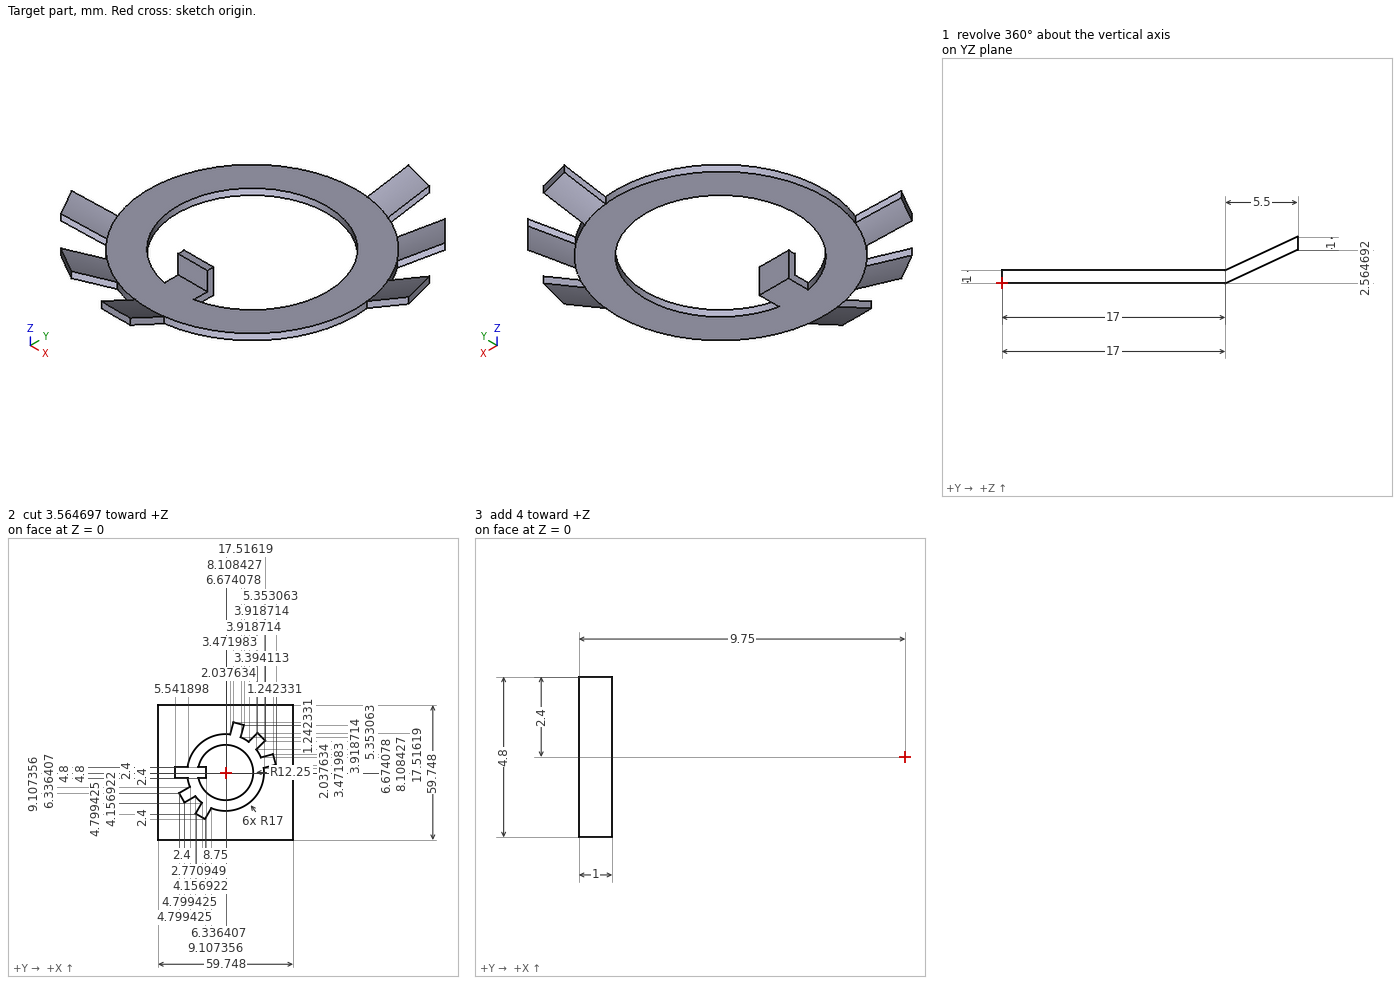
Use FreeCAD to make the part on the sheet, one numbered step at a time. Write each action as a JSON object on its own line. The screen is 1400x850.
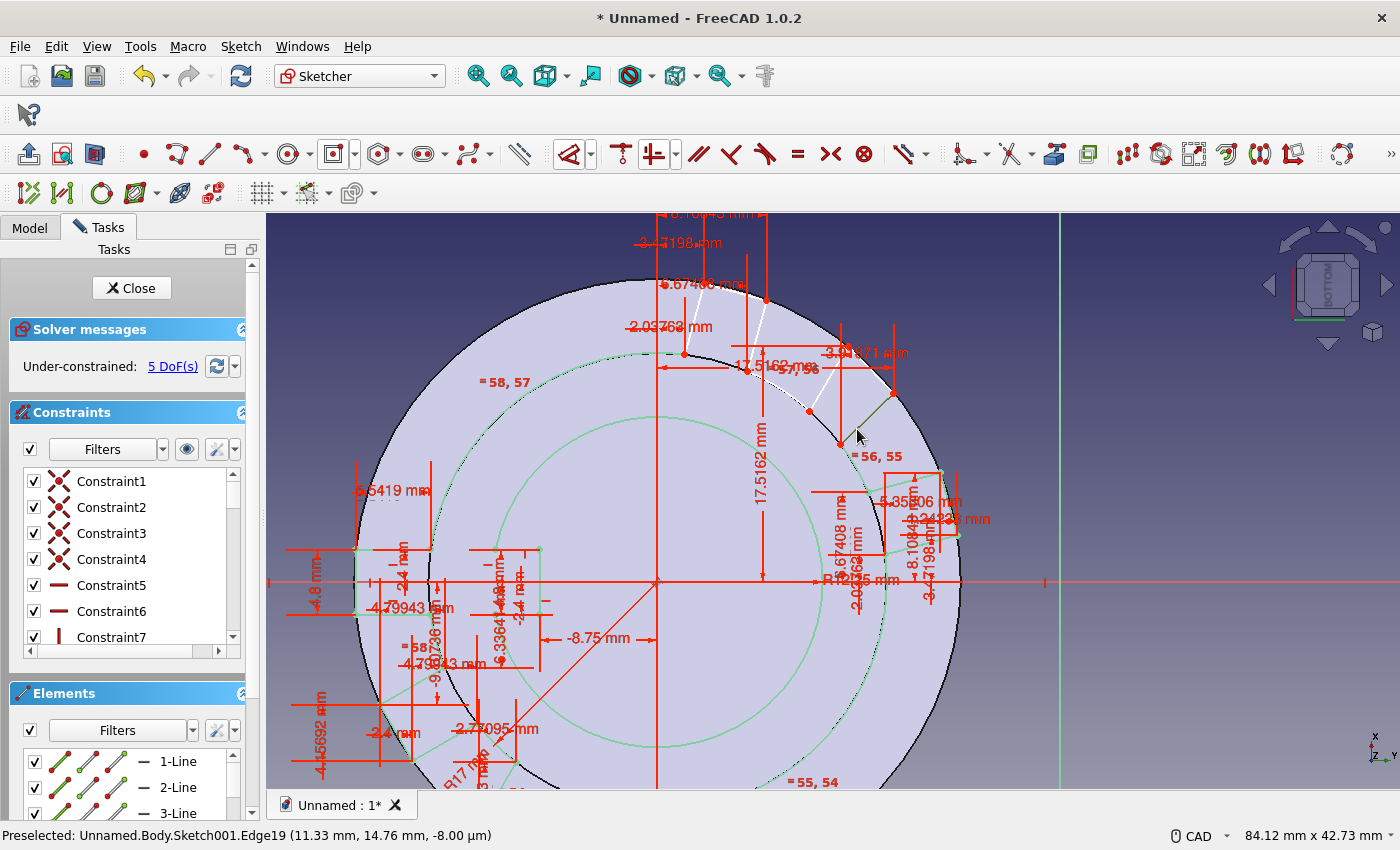
{"action": "key", "text": "i"}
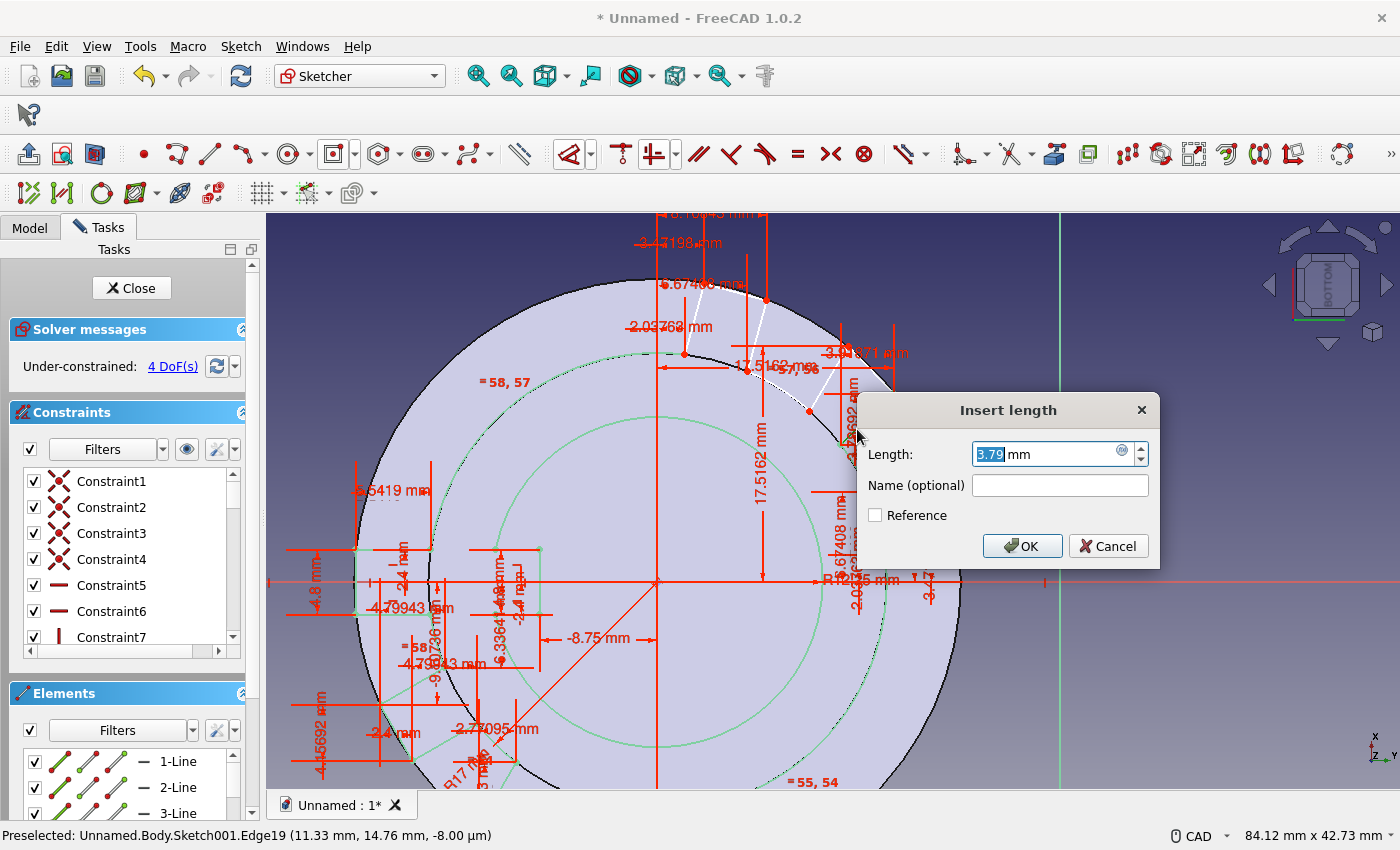
{"action": "type", "text": "3.918714"}
{"action": "key", "text": "Return"}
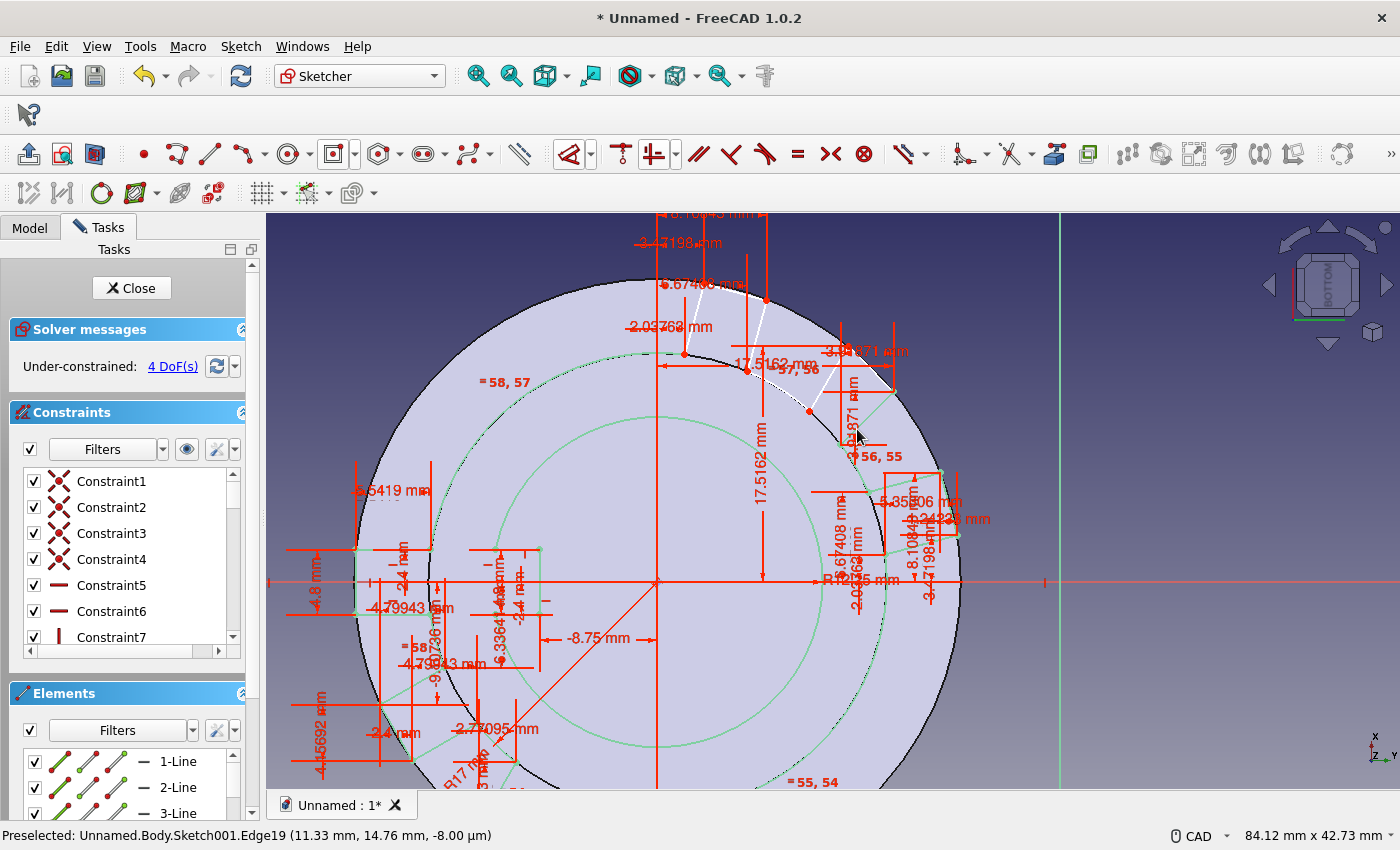
{"action": "left_click", "coordinate": [880, 378]}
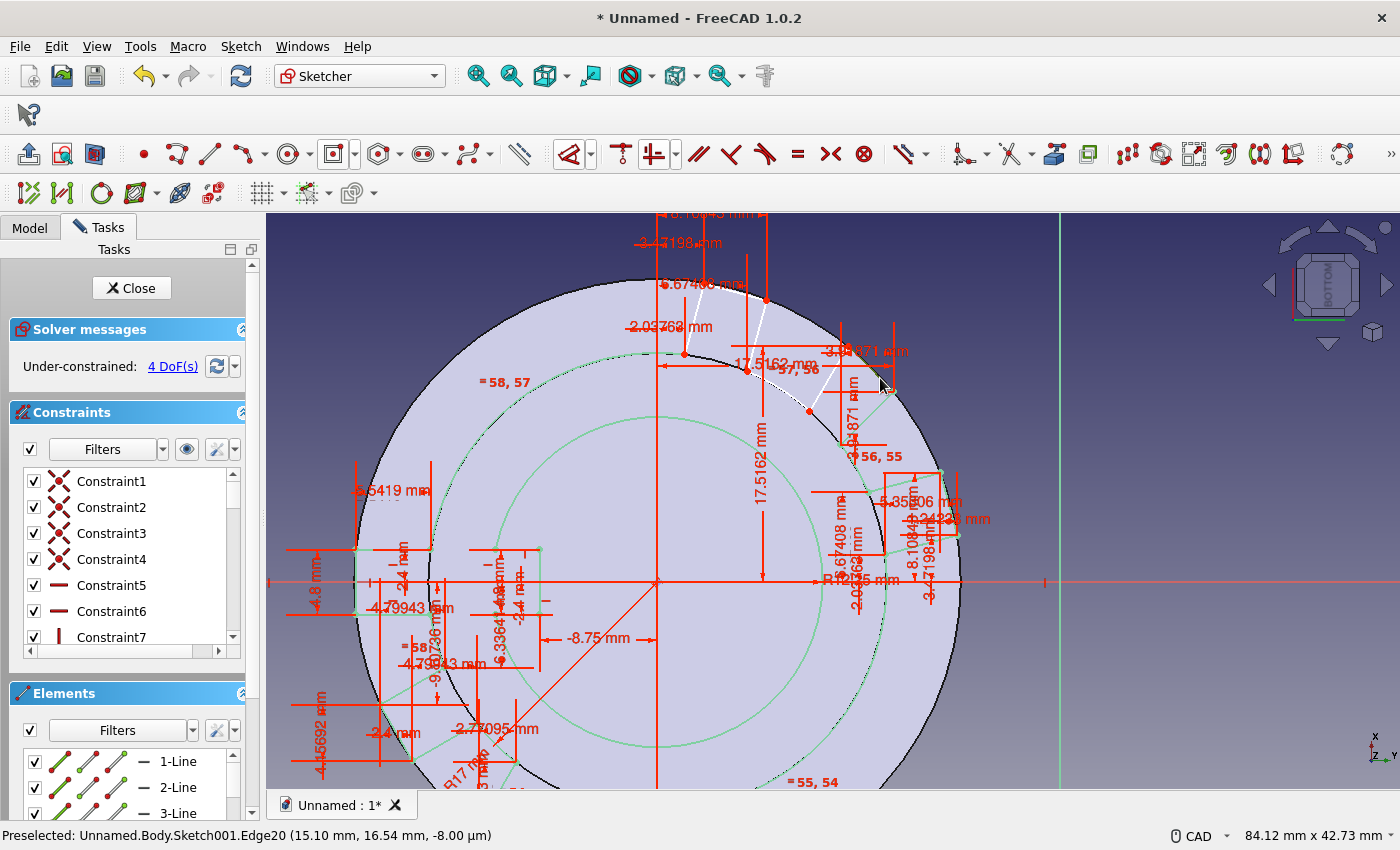
{"action": "left_click", "coordinate": [590, 154]}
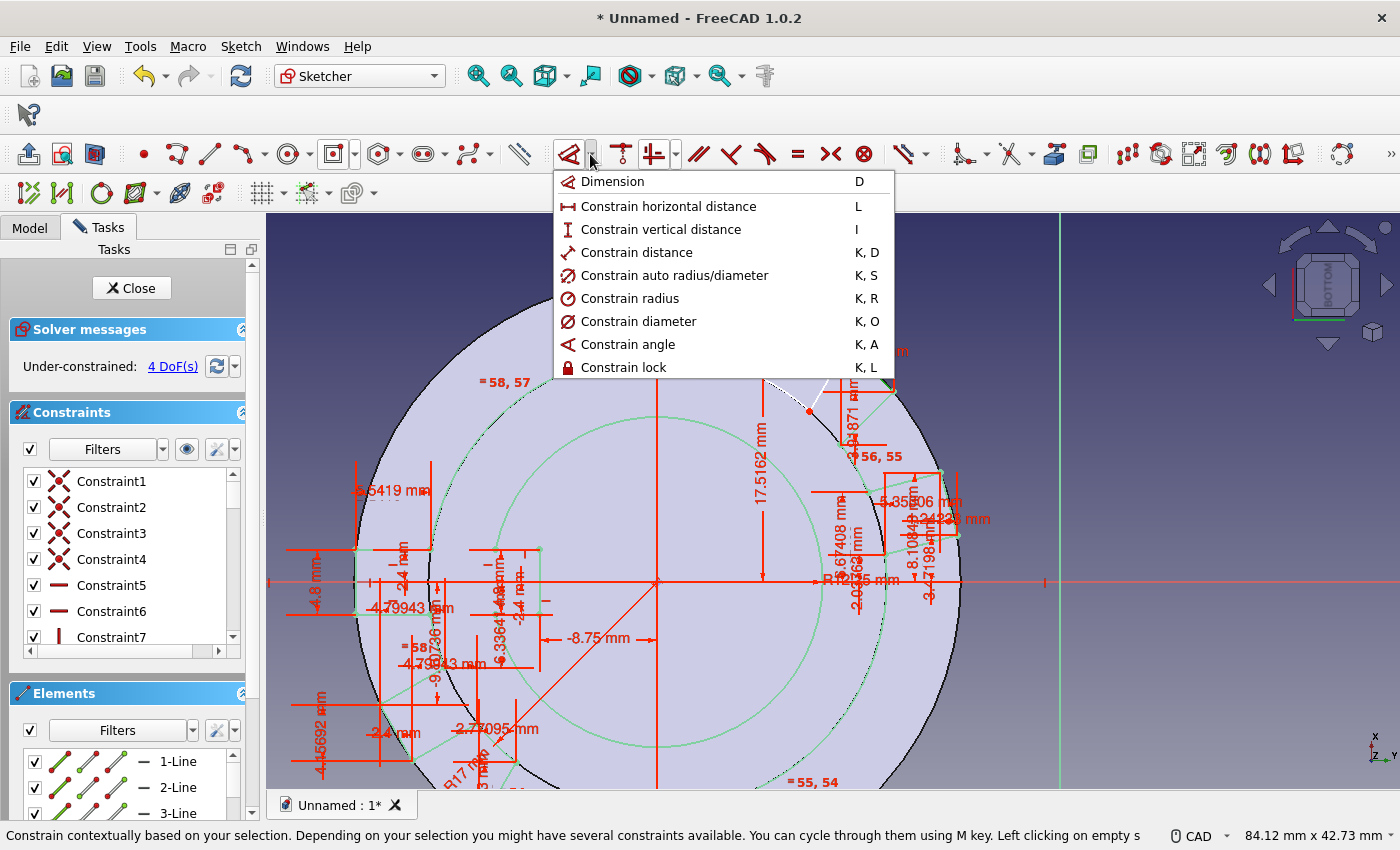
{"action": "left_click", "coordinate": [724, 206]}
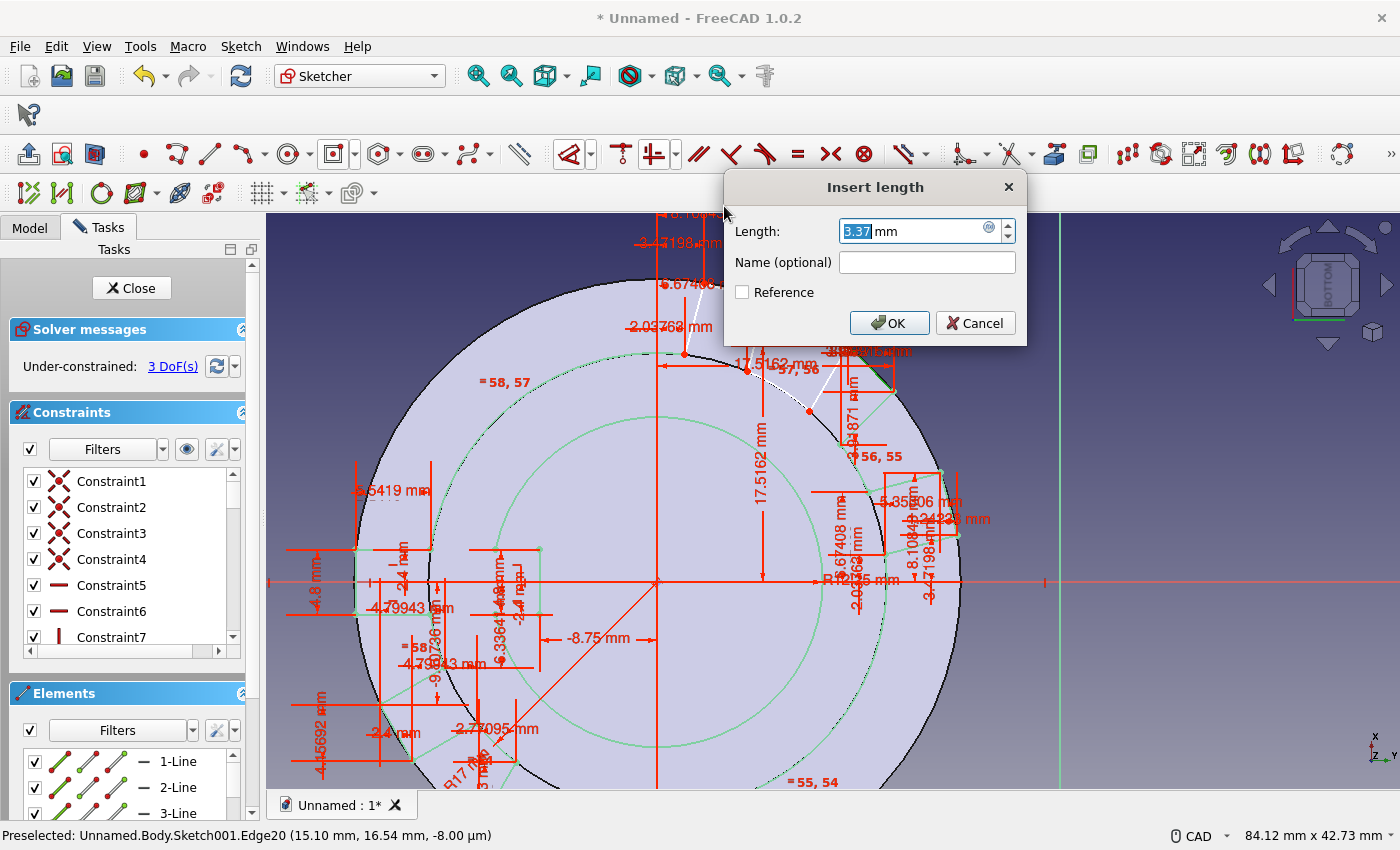
{"action": "type", "text": "3.394113"}
{"action": "key", "text": "Return"}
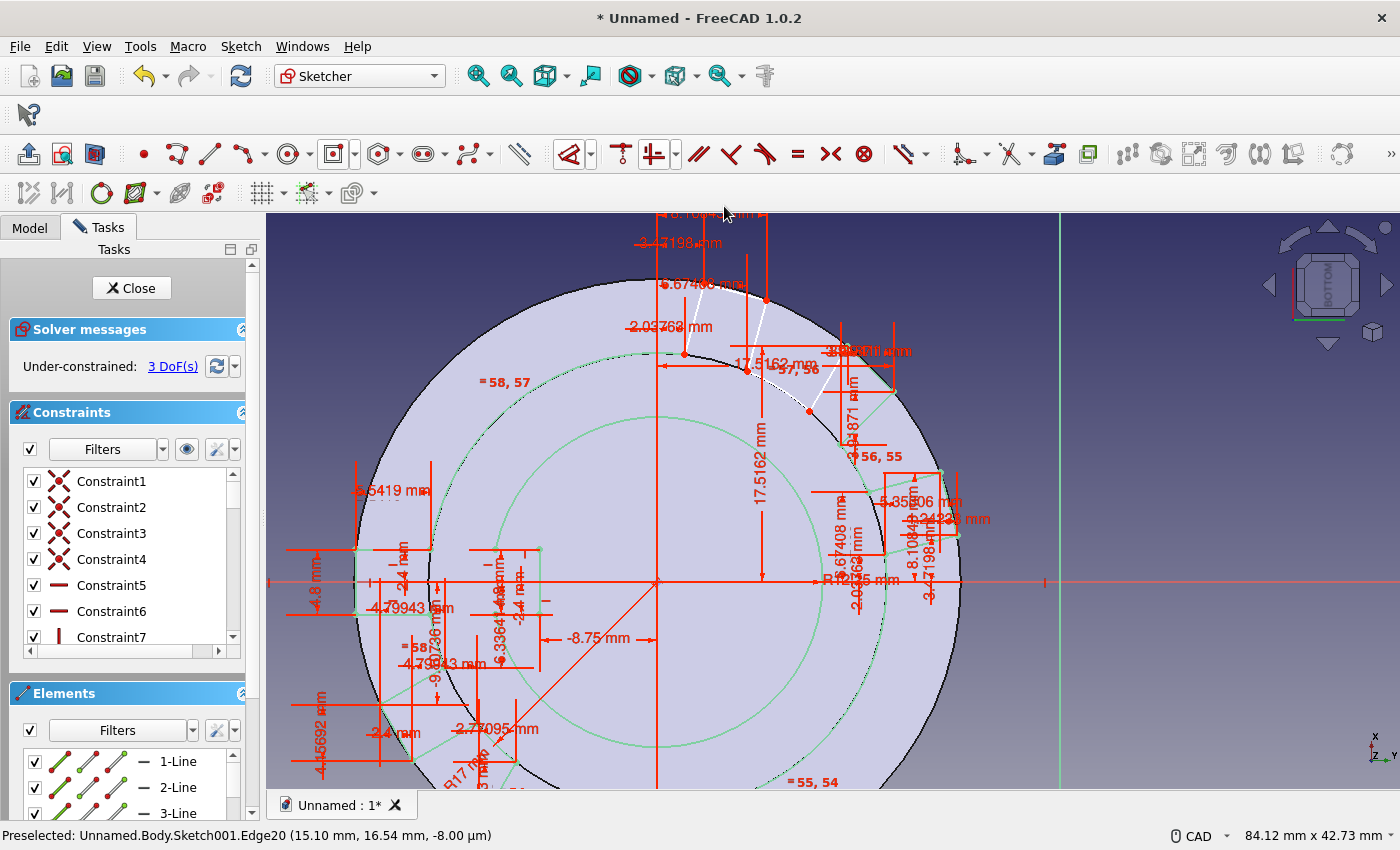
{"action": "left_click", "coordinate": [836, 366]}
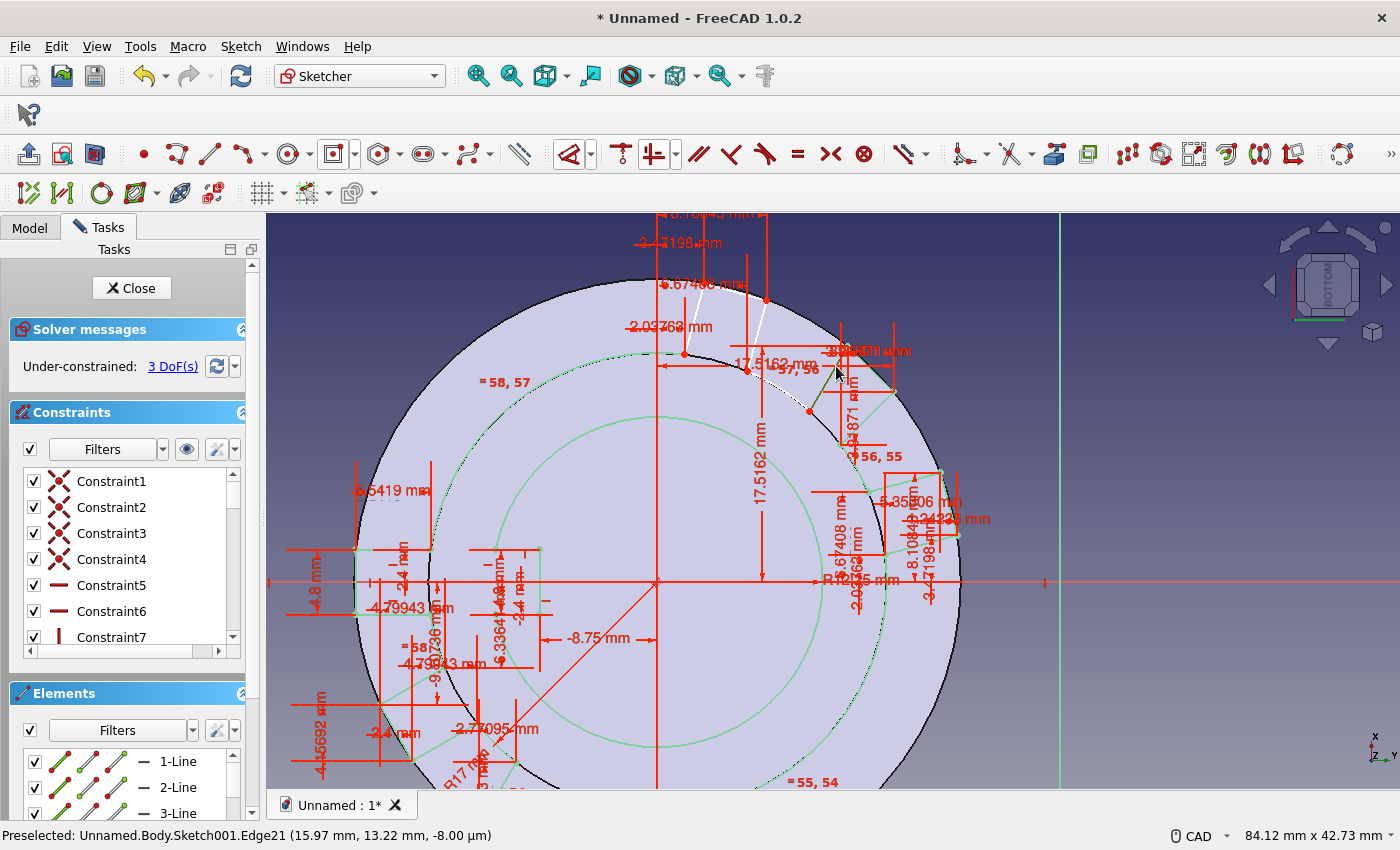
{"action": "key", "text": "l"}